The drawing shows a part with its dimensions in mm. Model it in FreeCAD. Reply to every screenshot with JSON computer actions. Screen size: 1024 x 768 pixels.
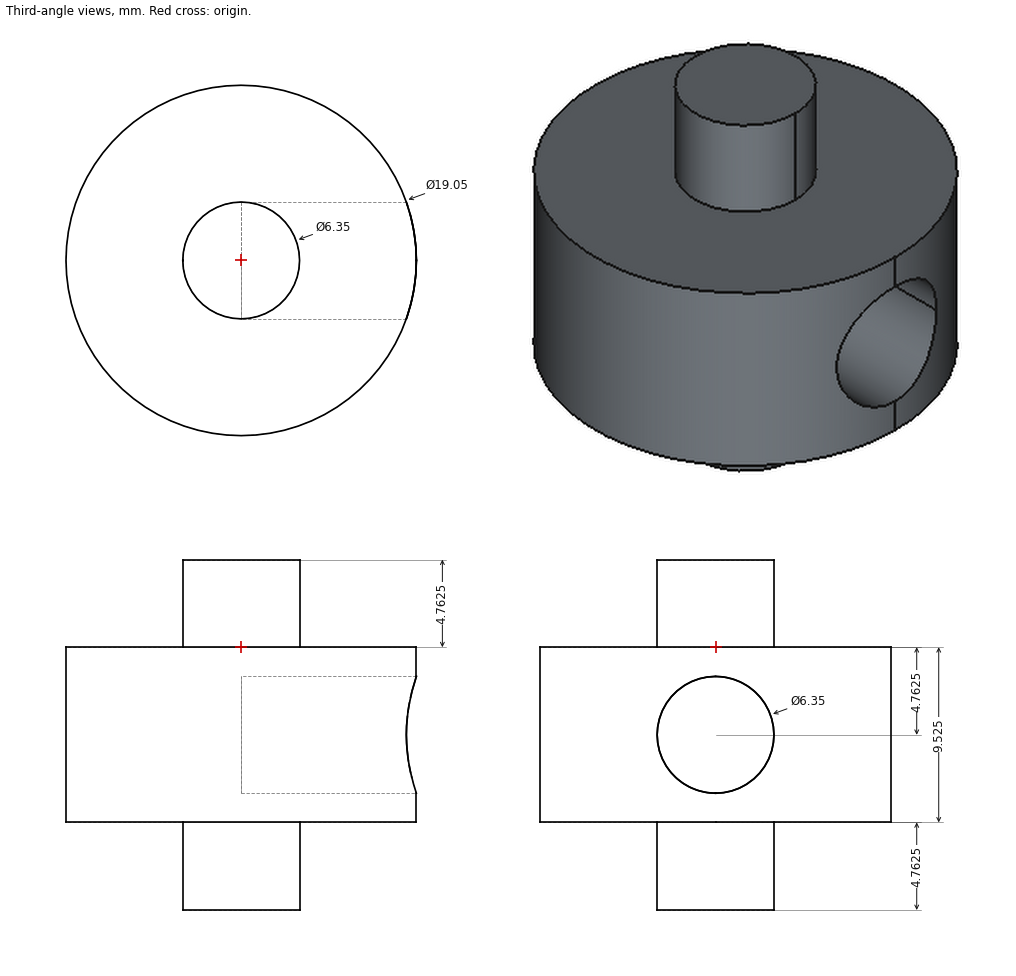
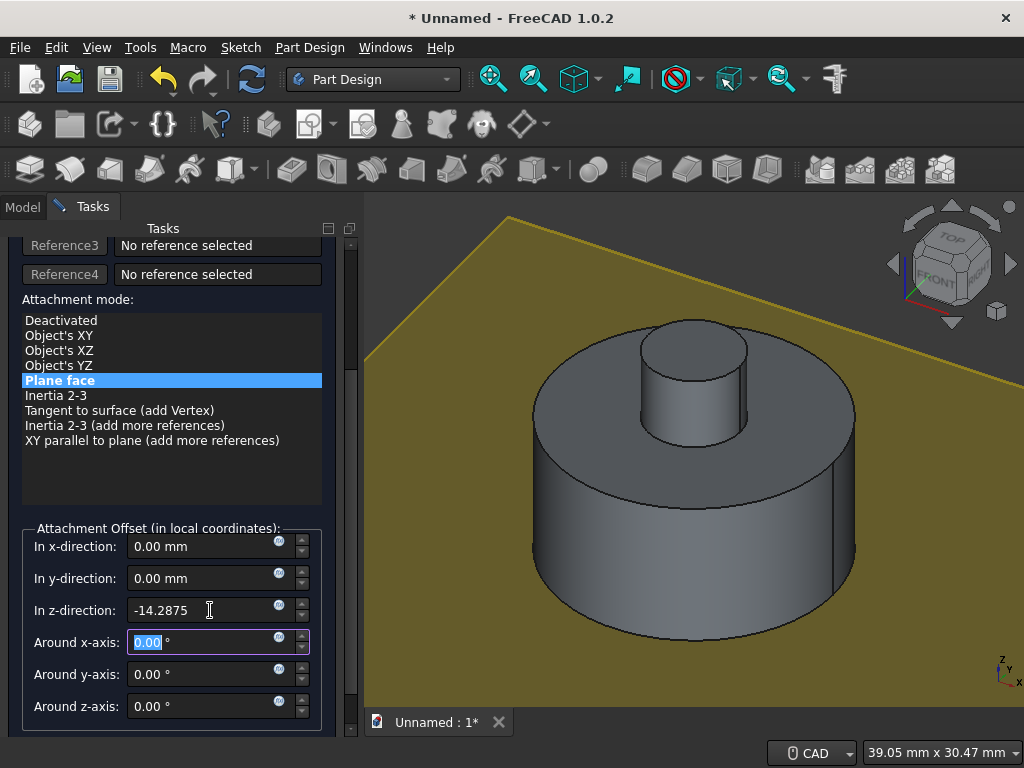
{"action": "scroll", "coordinate": [351, 487], "scroll_direction": "up", "scroll_amount": 4}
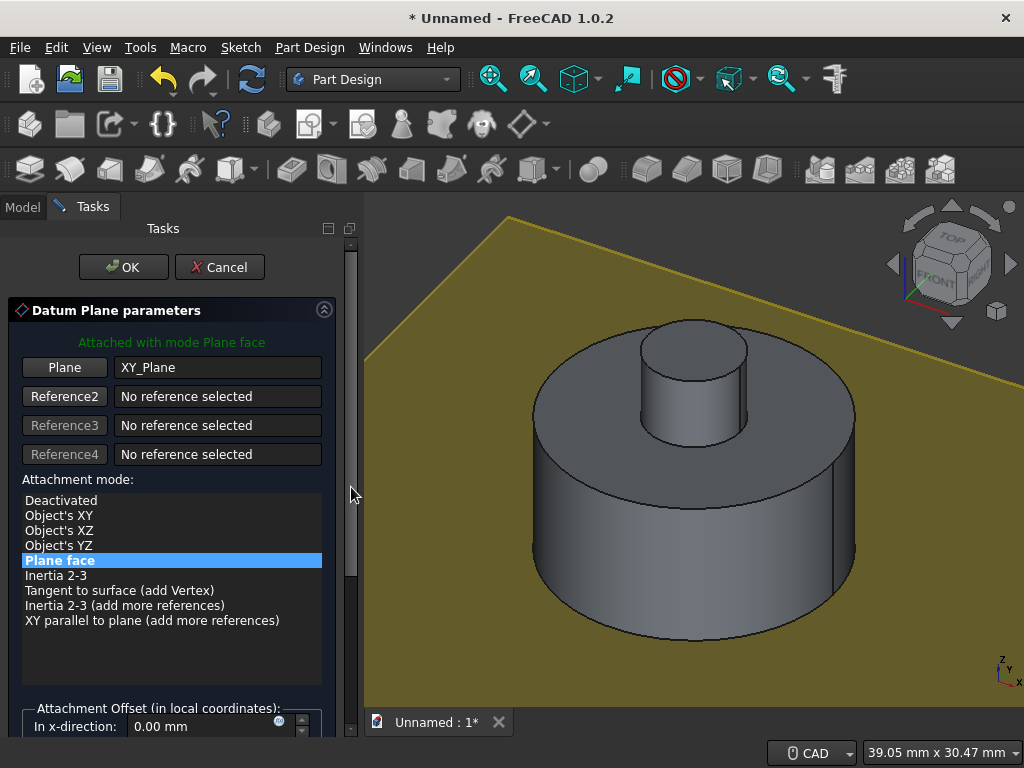
{"action": "left_click", "coordinate": [124, 267]}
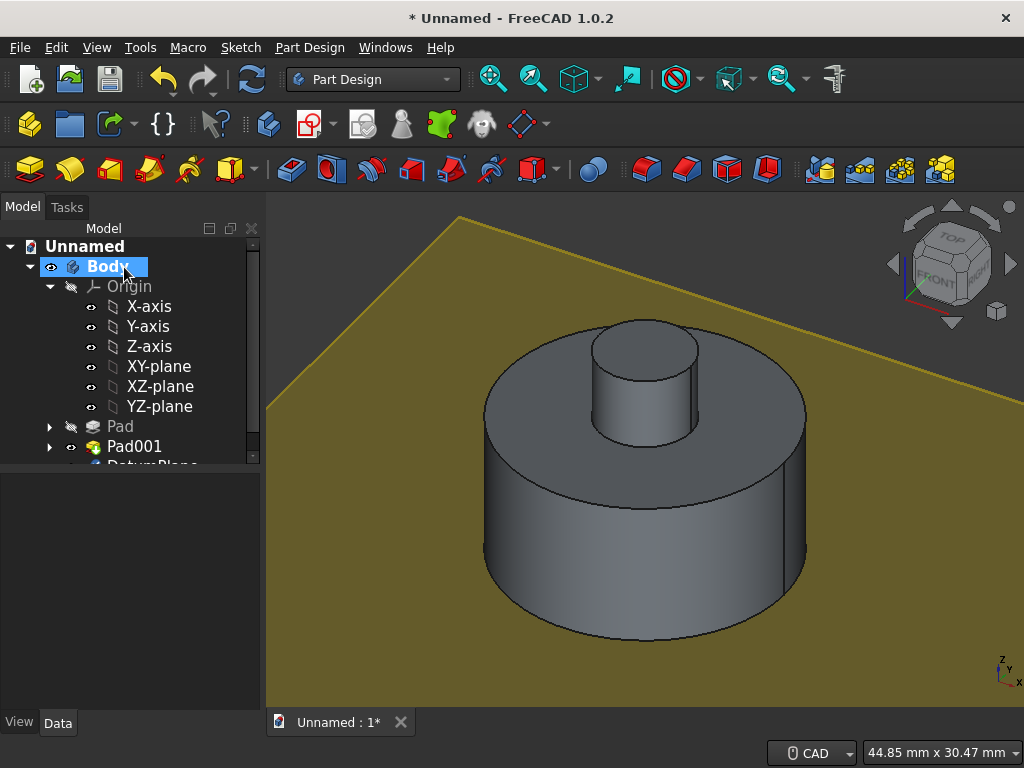
{"action": "scroll", "coordinate": [100, 342], "scroll_direction": "down", "scroll_amount": 3}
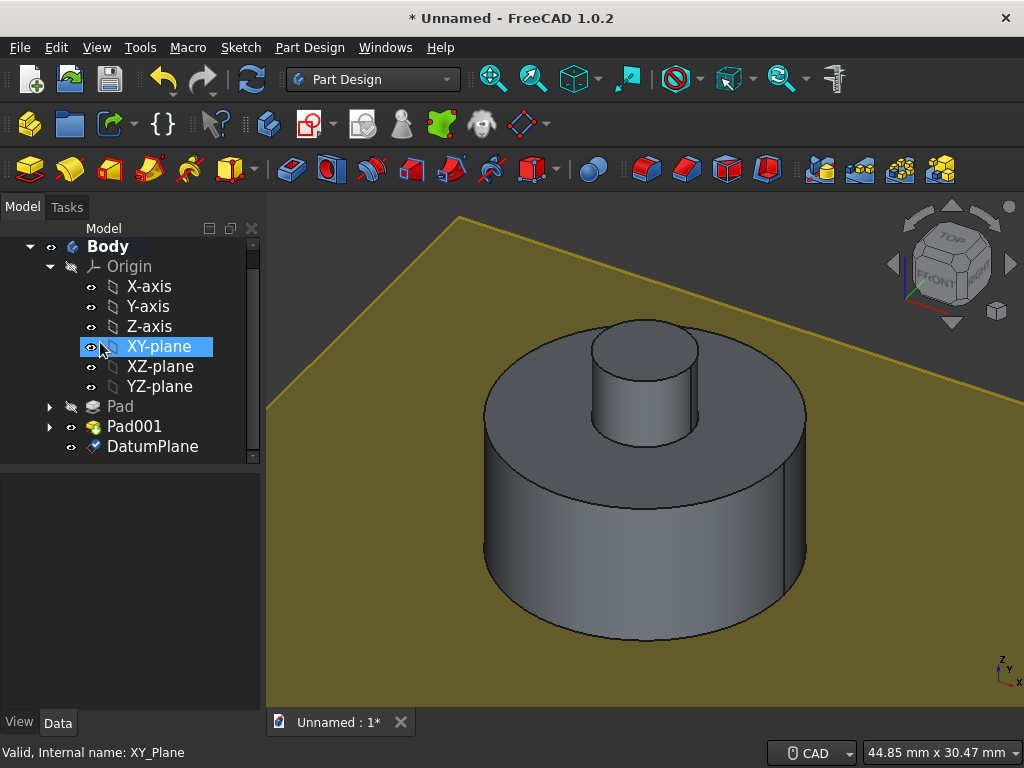
{"action": "left_click", "coordinate": [116, 447]}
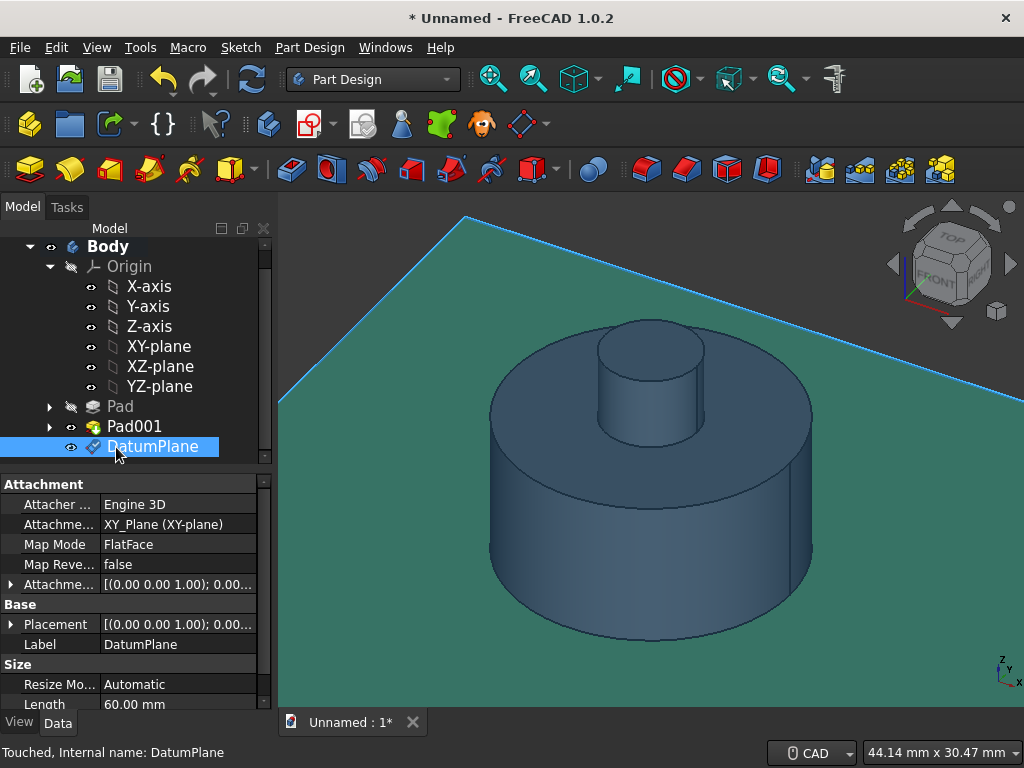
{"action": "left_click", "coordinate": [310, 124]}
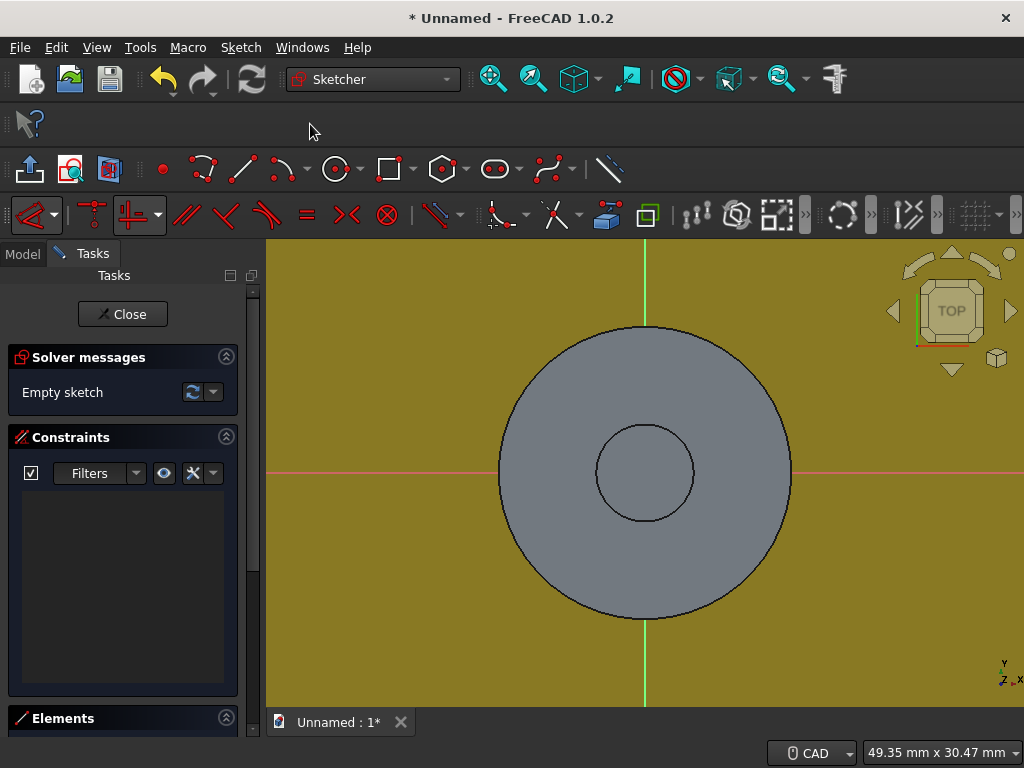
{"action": "left_click", "coordinate": [110, 170]}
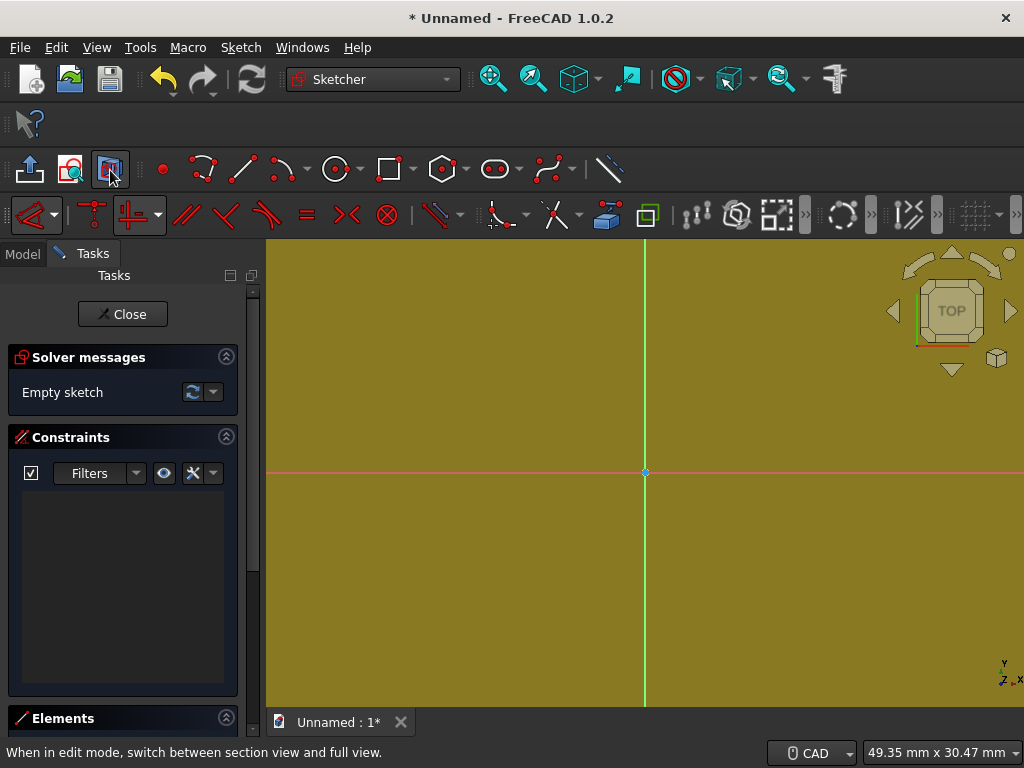
{"action": "scroll", "coordinate": [685, 473], "scroll_direction": "up", "scroll_amount": 5}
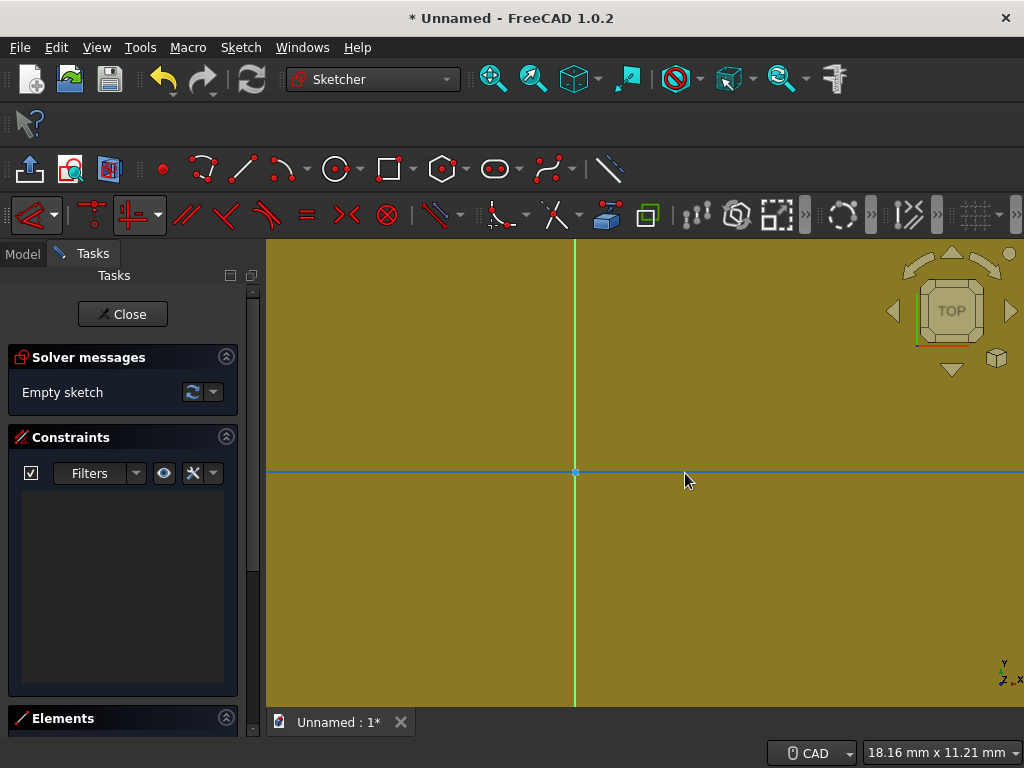
{"action": "left_click", "coordinate": [336, 170]}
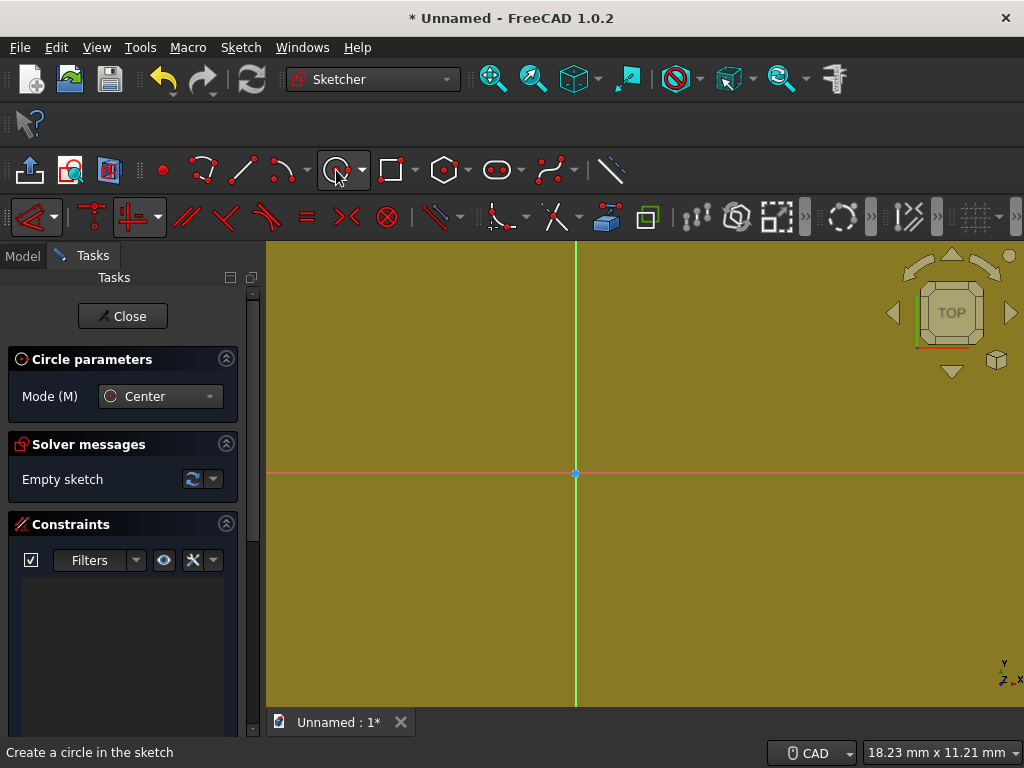
{"action": "left_click", "coordinate": [576, 473]}
{"action": "left_click", "coordinate": [669, 380]}
{"action": "key", "text": "Escape"}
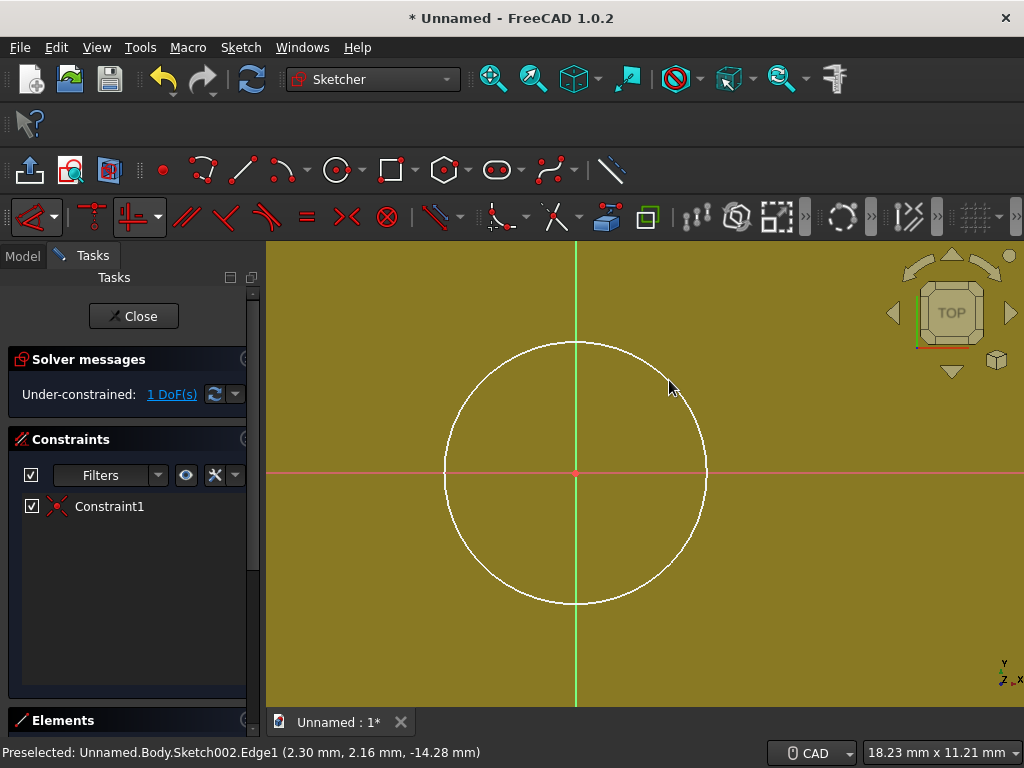
{"action": "left_click", "coordinate": [668, 380]}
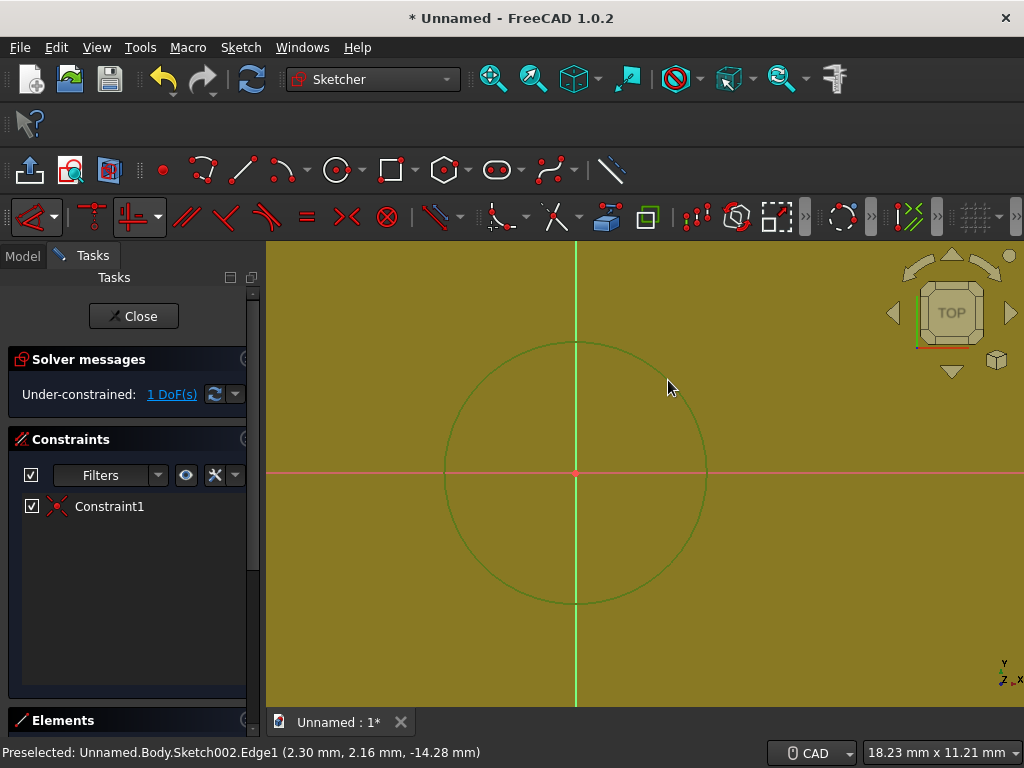
{"action": "left_click", "coordinate": [56, 218]}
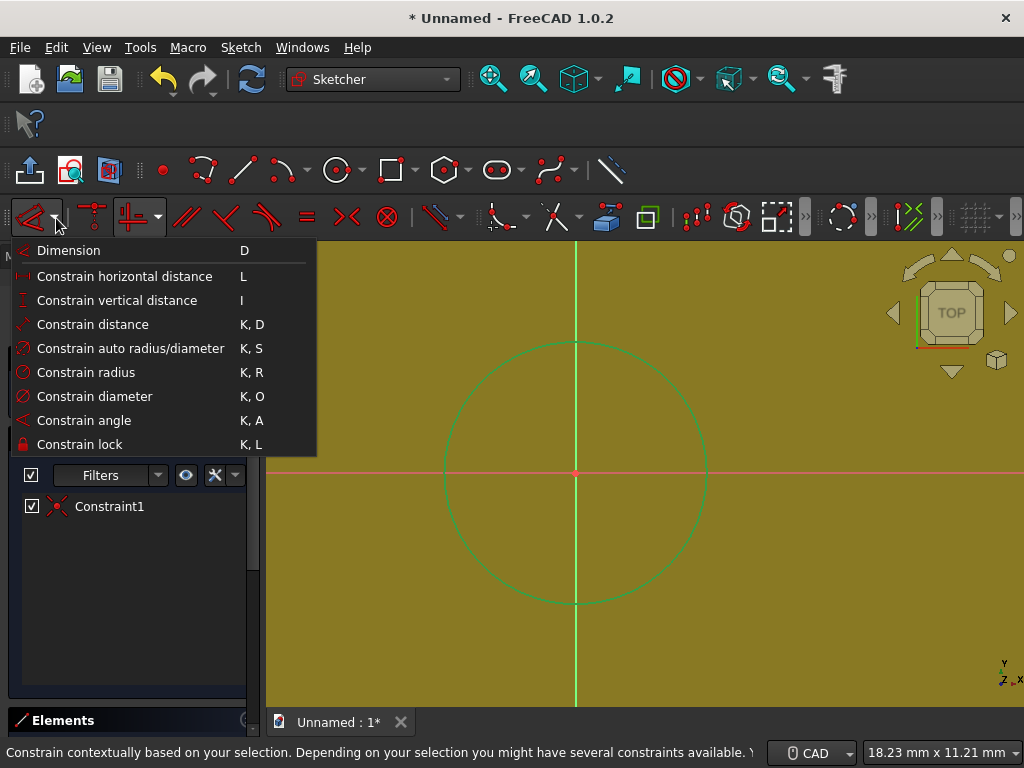
{"action": "left_click", "coordinate": [164, 396]}